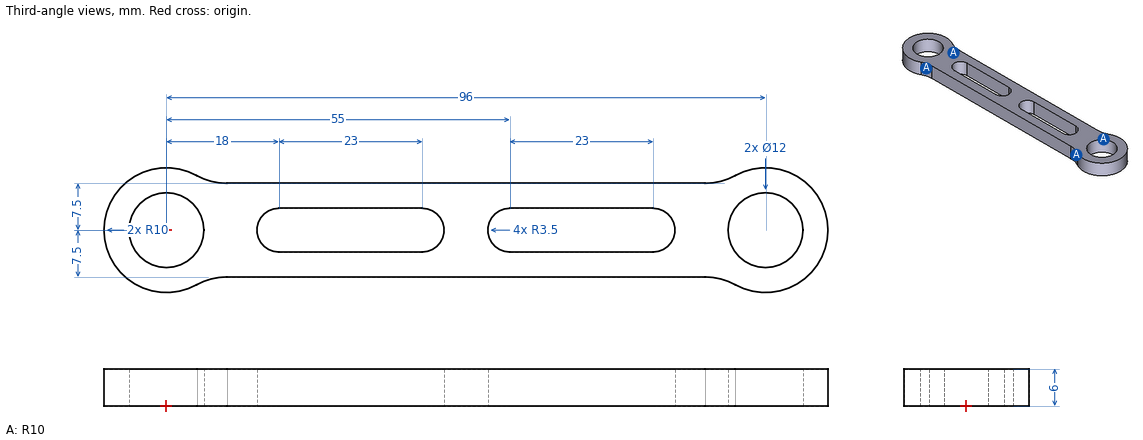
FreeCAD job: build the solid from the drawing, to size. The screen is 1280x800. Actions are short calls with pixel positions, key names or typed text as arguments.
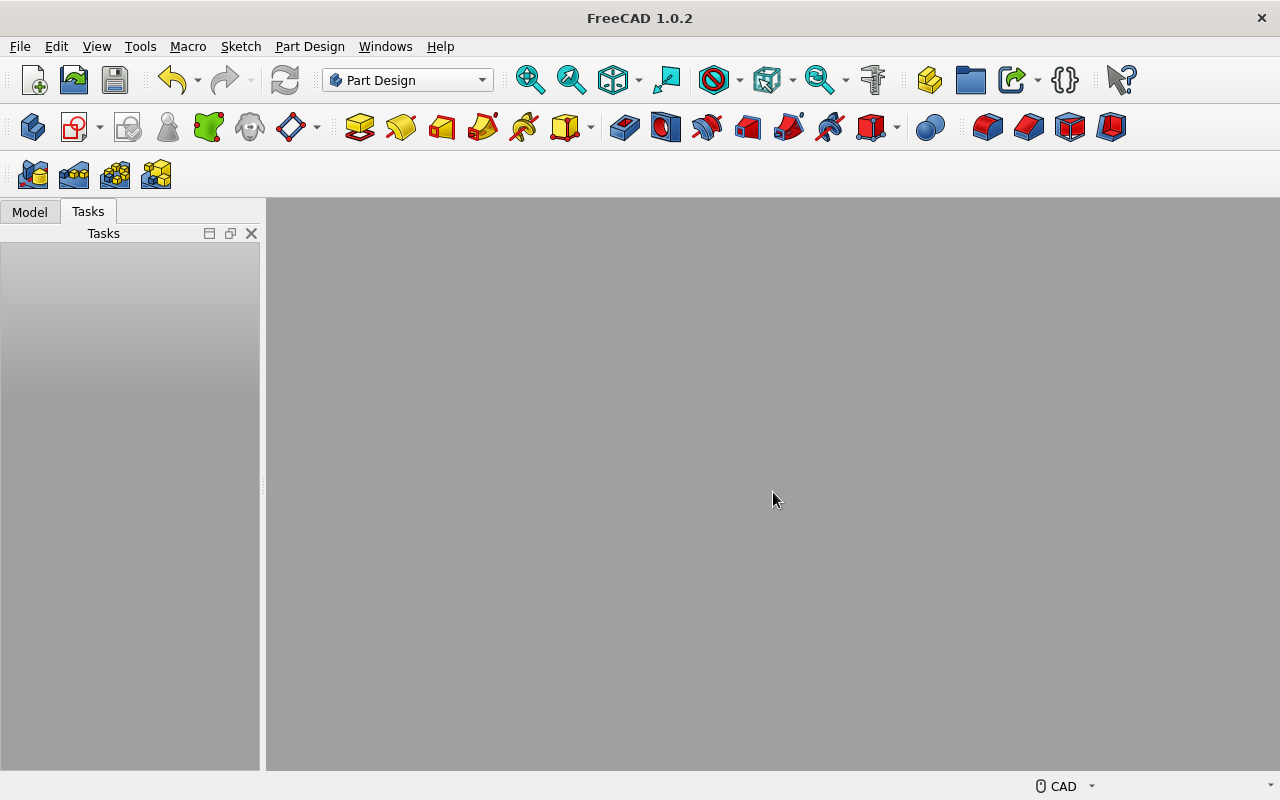
click(33, 80)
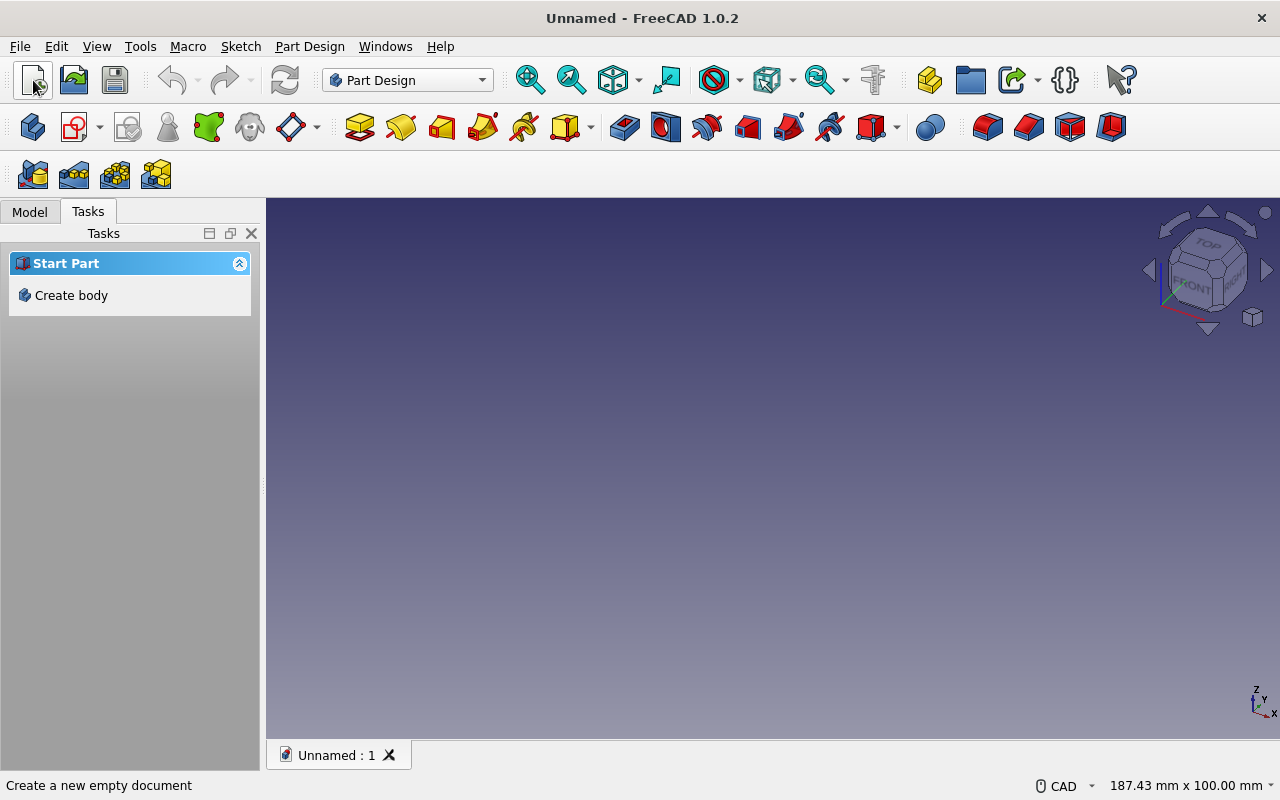
click(74, 128)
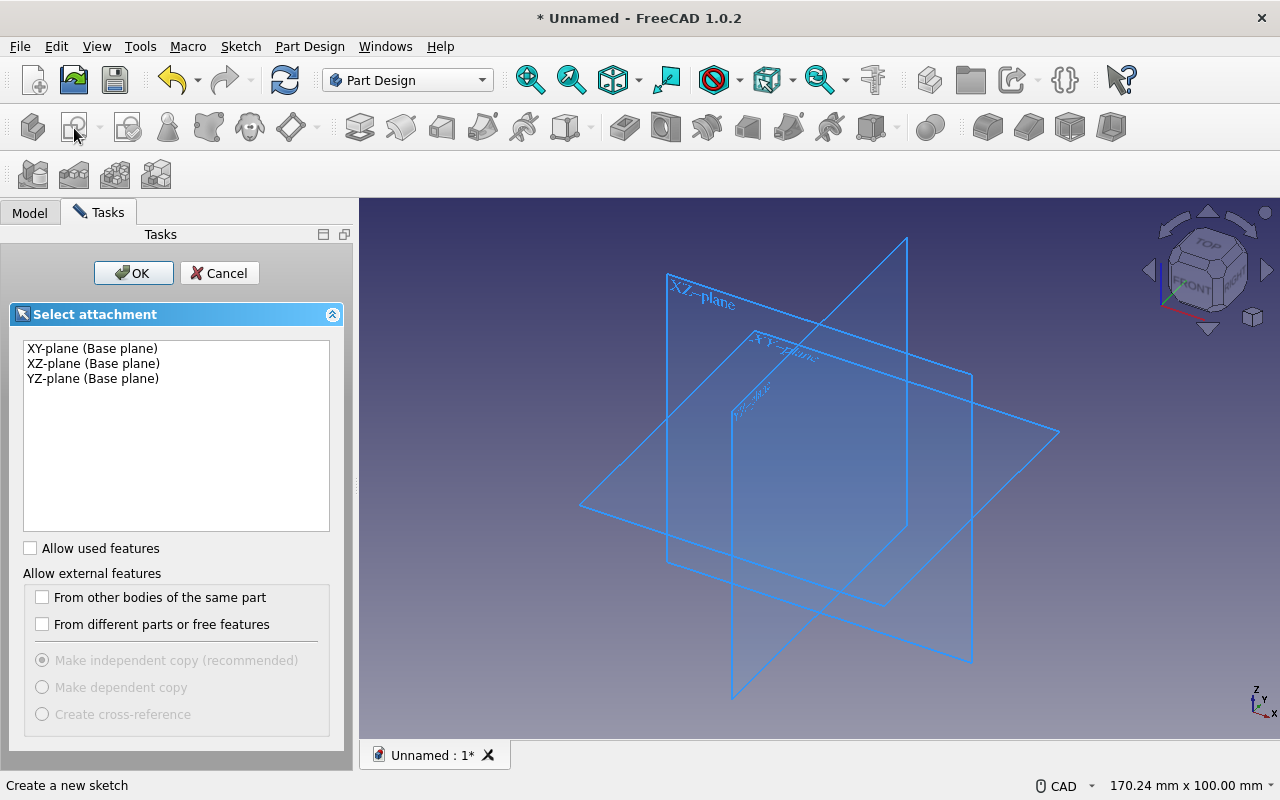
click(84, 348)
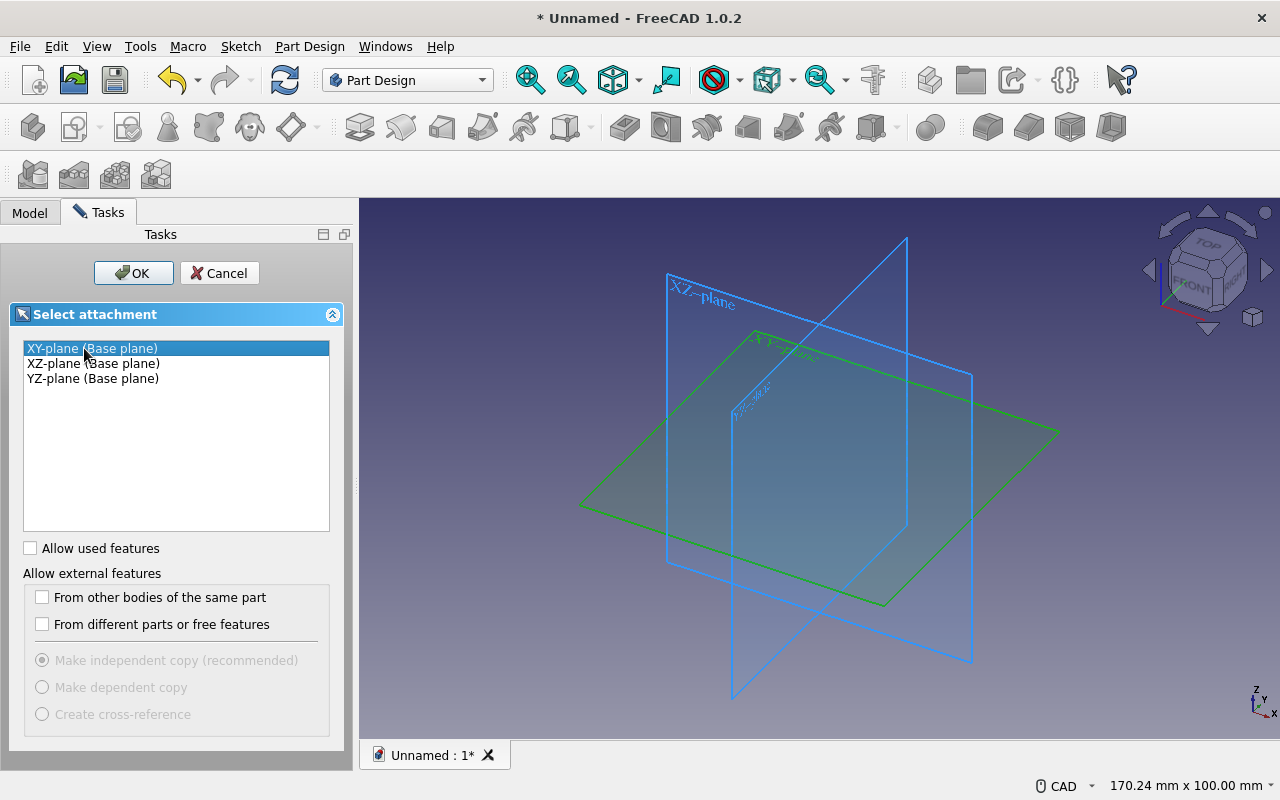
click(134, 273)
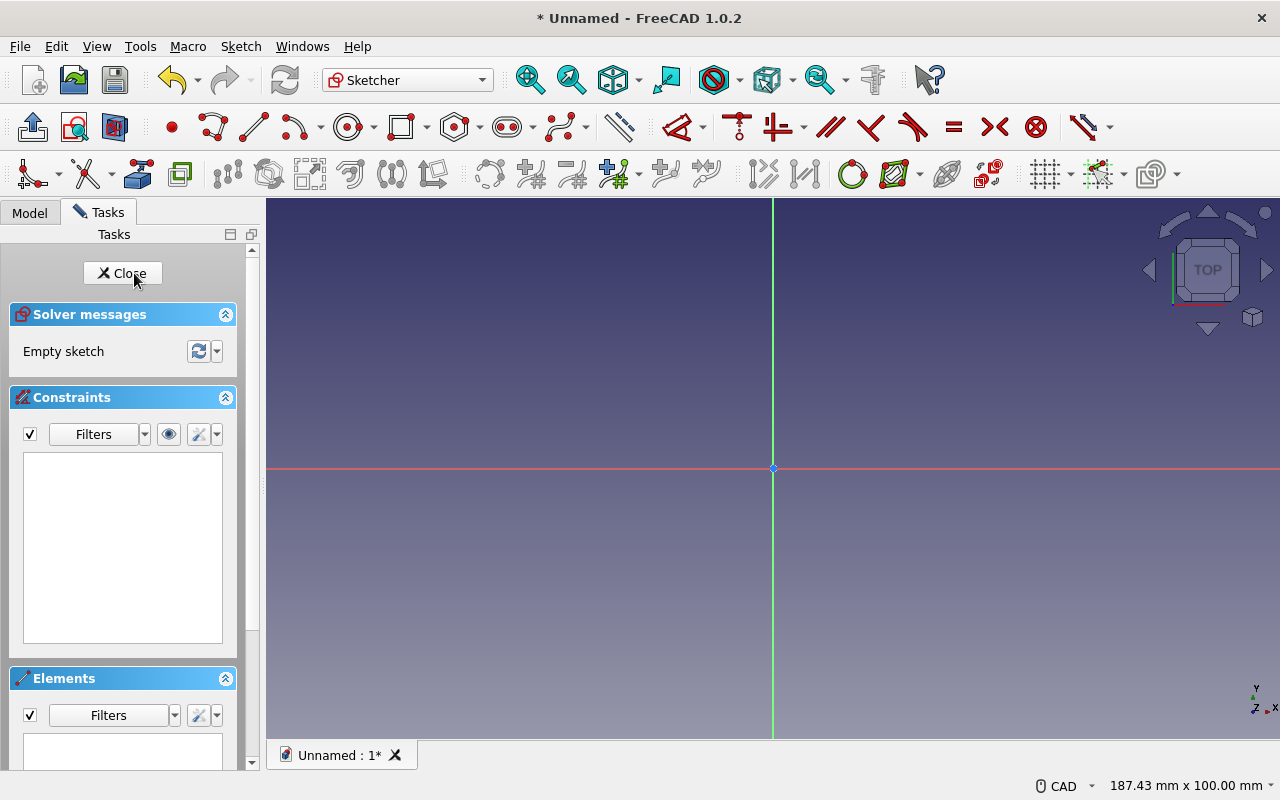
scroll(294, 468, down, 2)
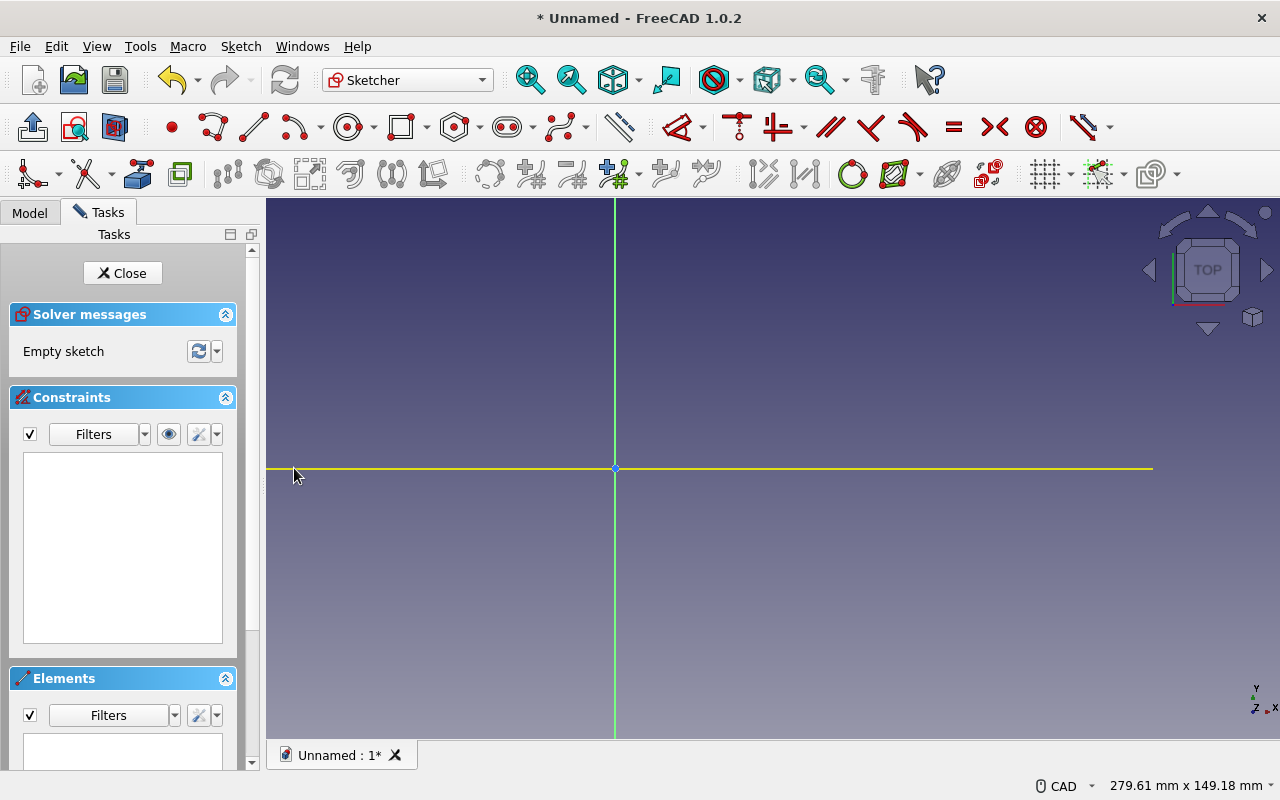
scroll(961, 469, up, 2)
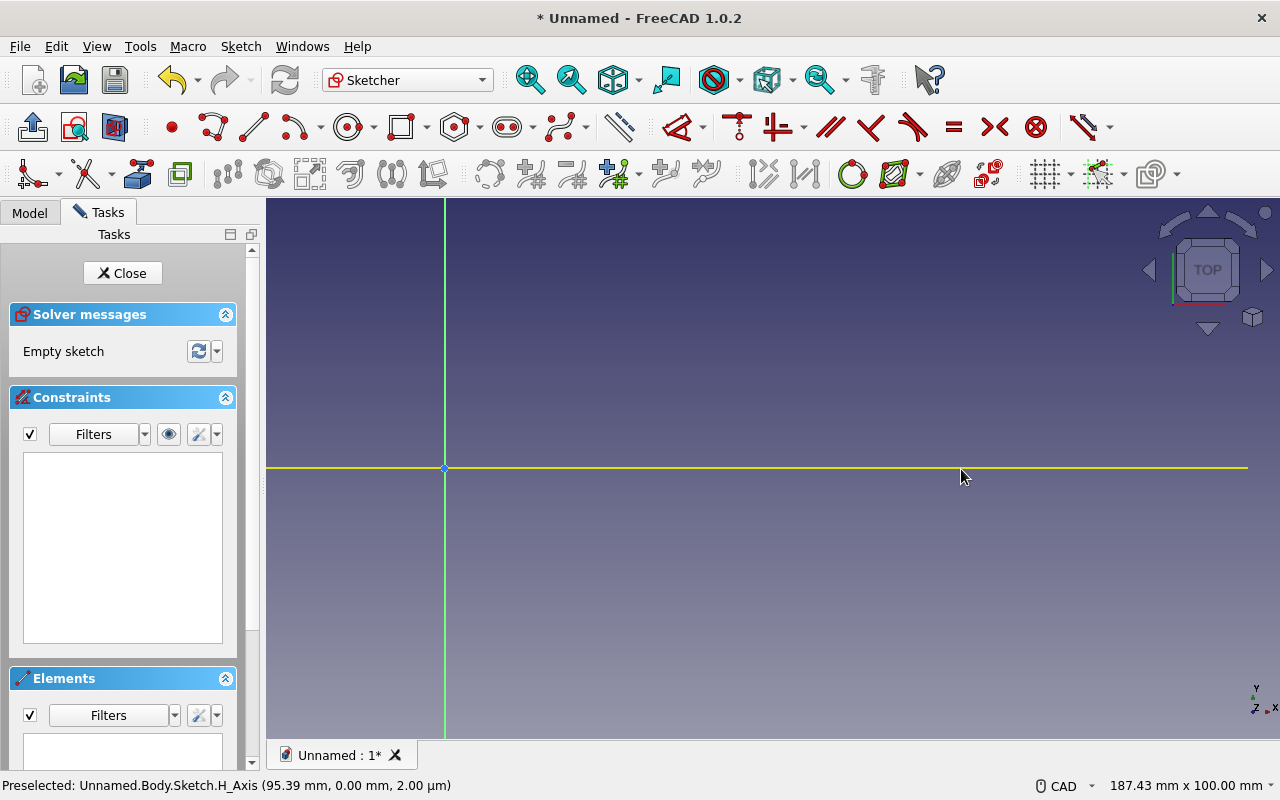
click(254, 128)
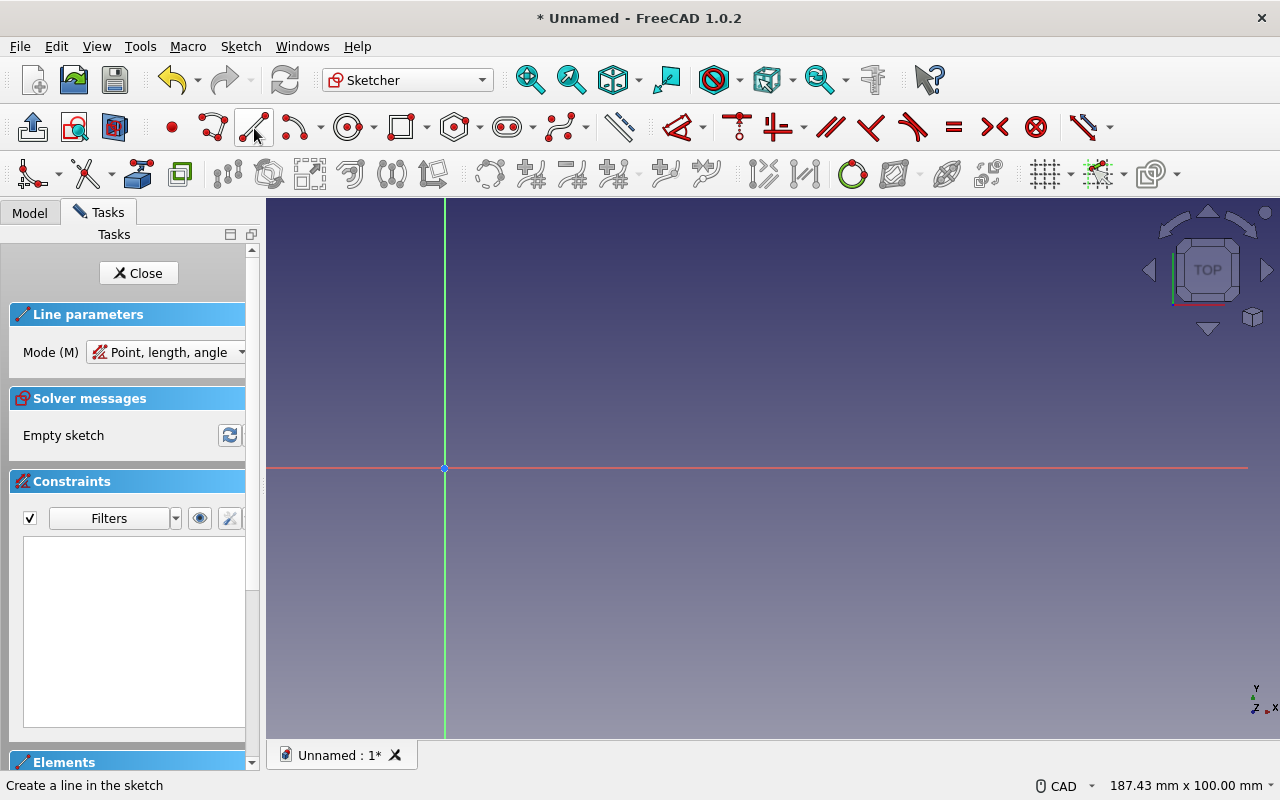
click(928, 427)
click(480, 427)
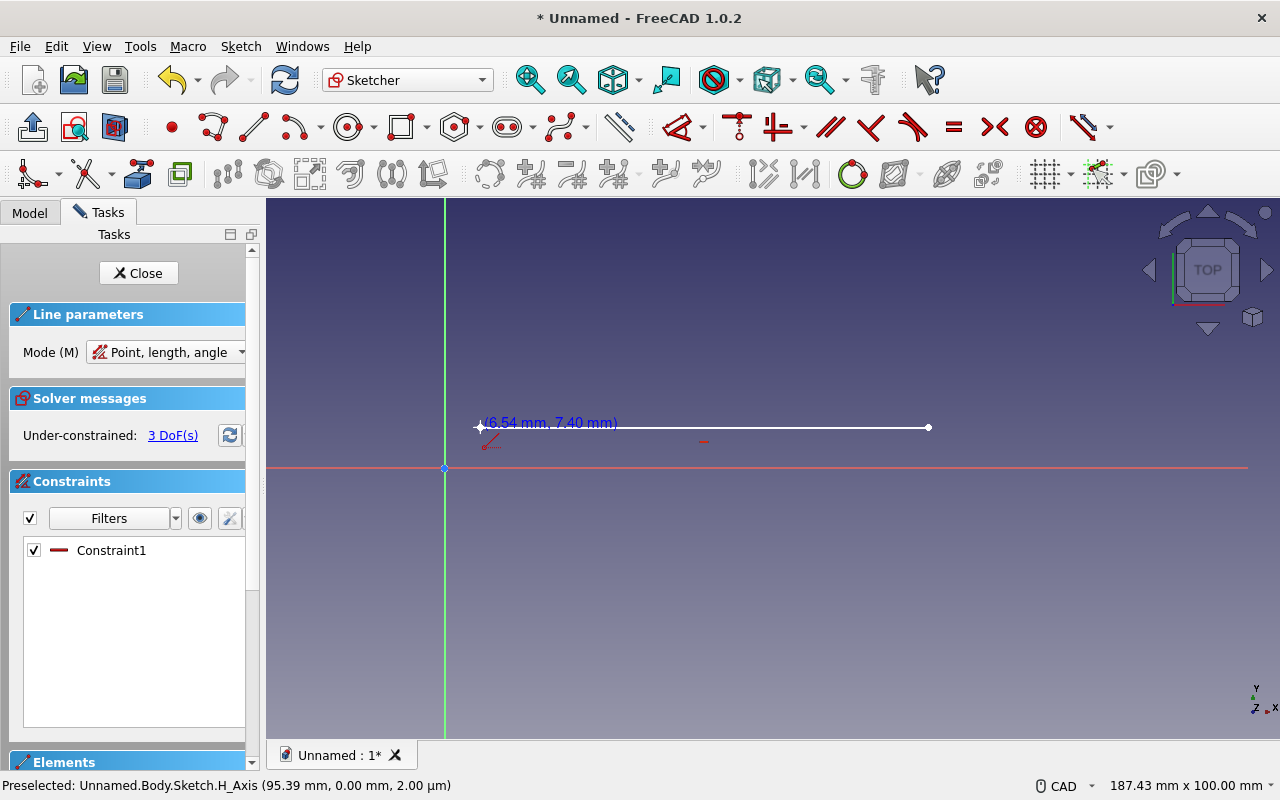
click(480, 509)
click(928, 509)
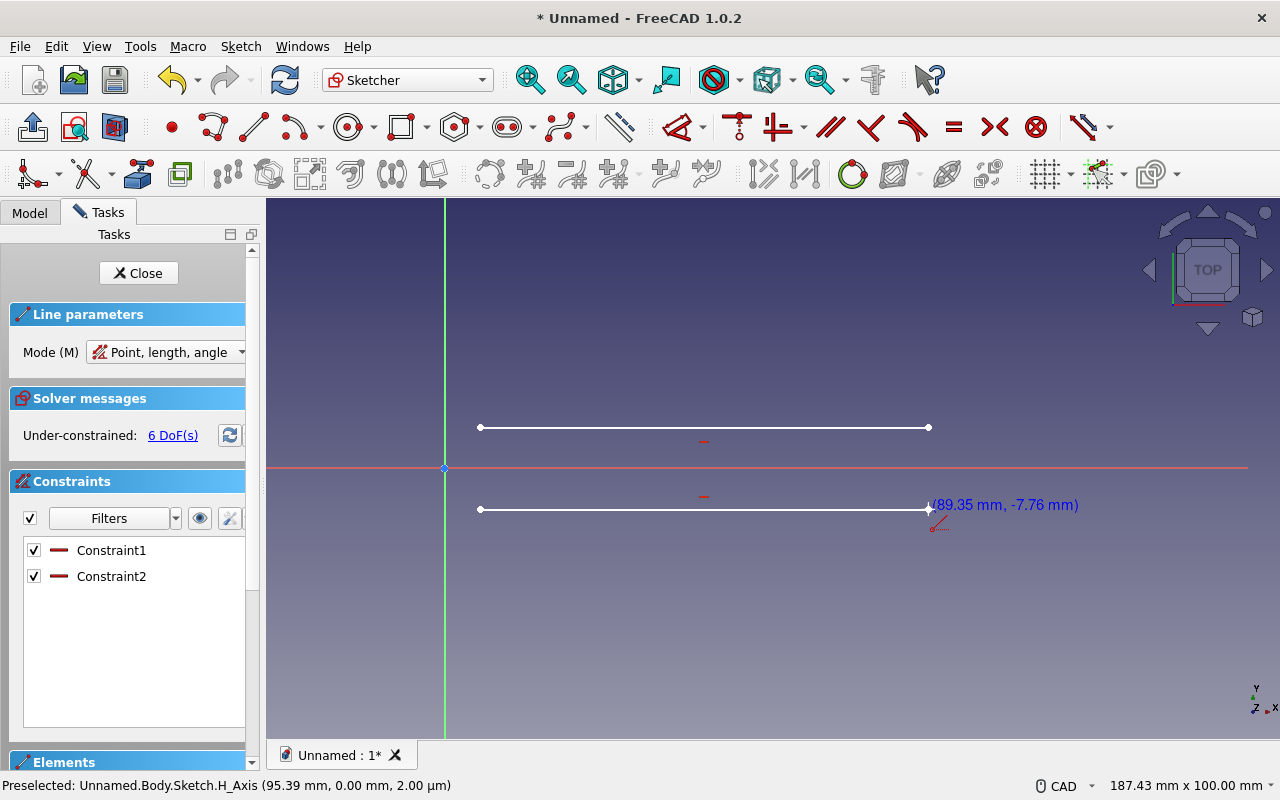
click(320, 128)